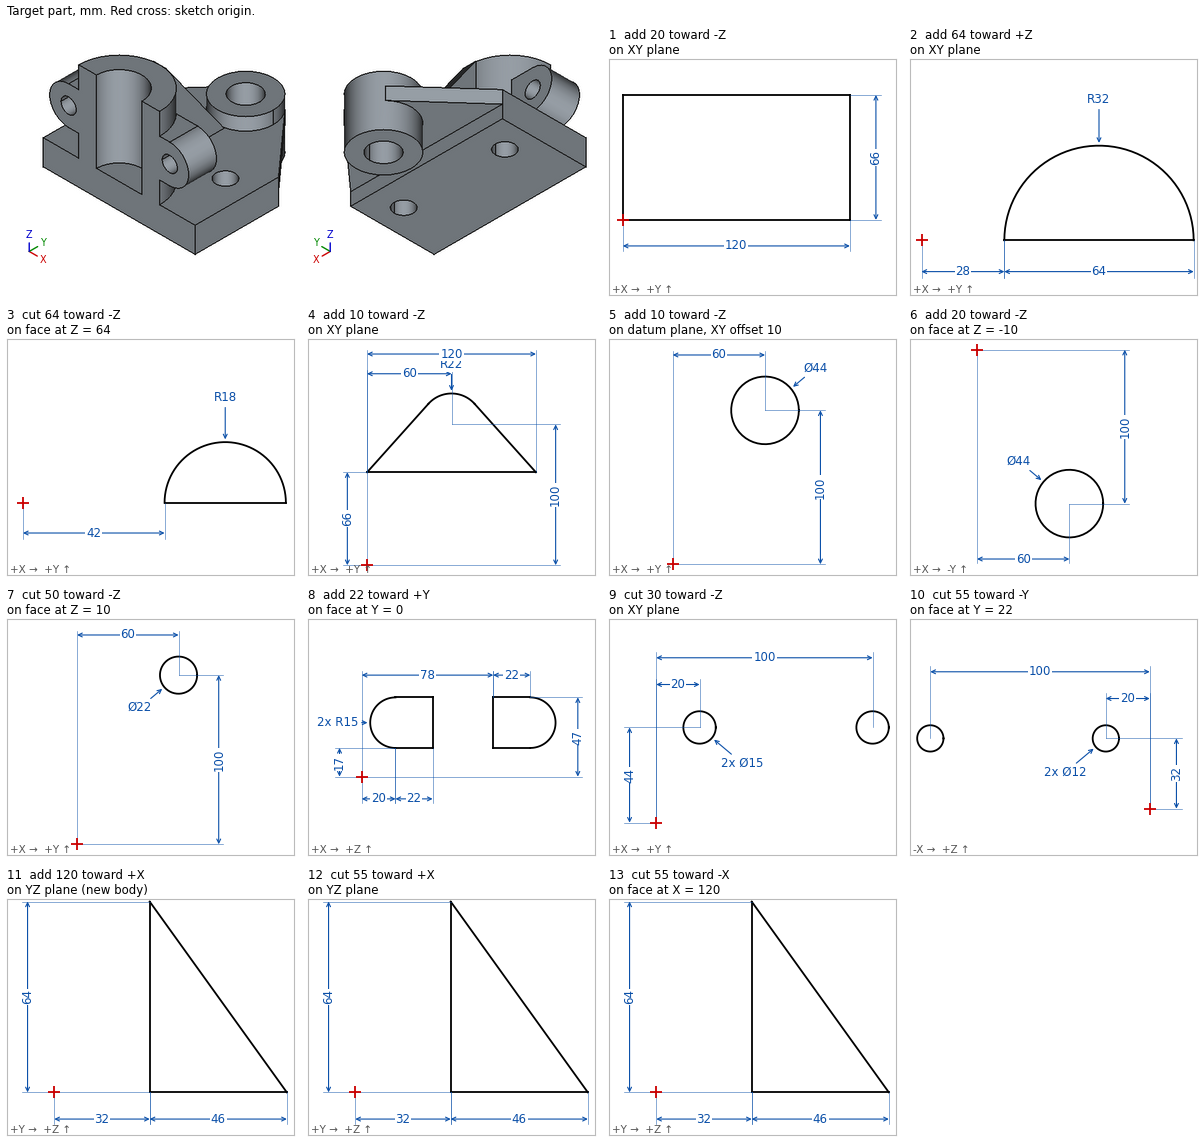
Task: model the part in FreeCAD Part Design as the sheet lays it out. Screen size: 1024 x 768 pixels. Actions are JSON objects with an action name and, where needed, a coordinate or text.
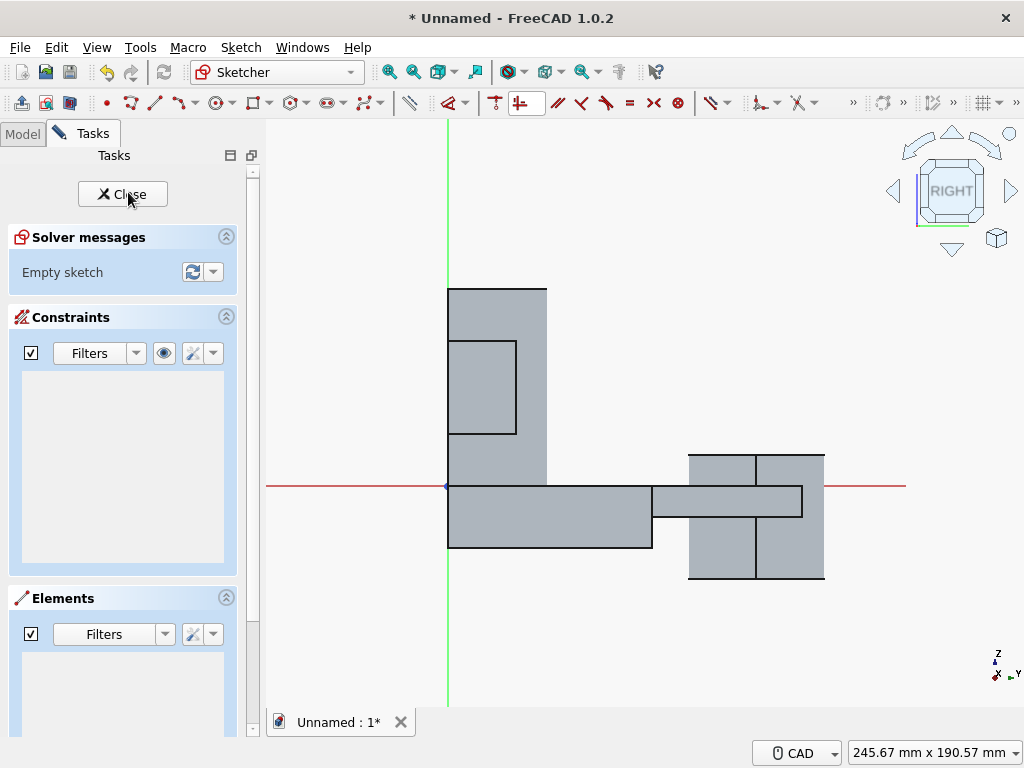
{"action": "scroll", "coordinate": [558, 356], "scroll_direction": "up", "scroll_amount": 3}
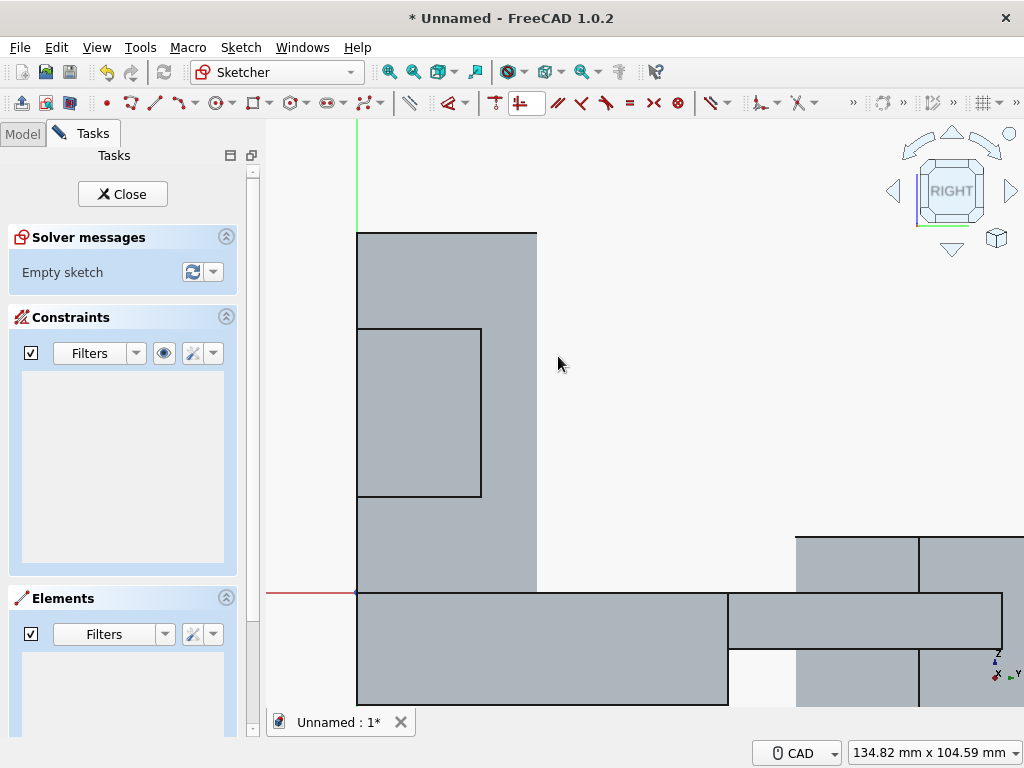
{"action": "left_click", "coordinate": [132, 104]}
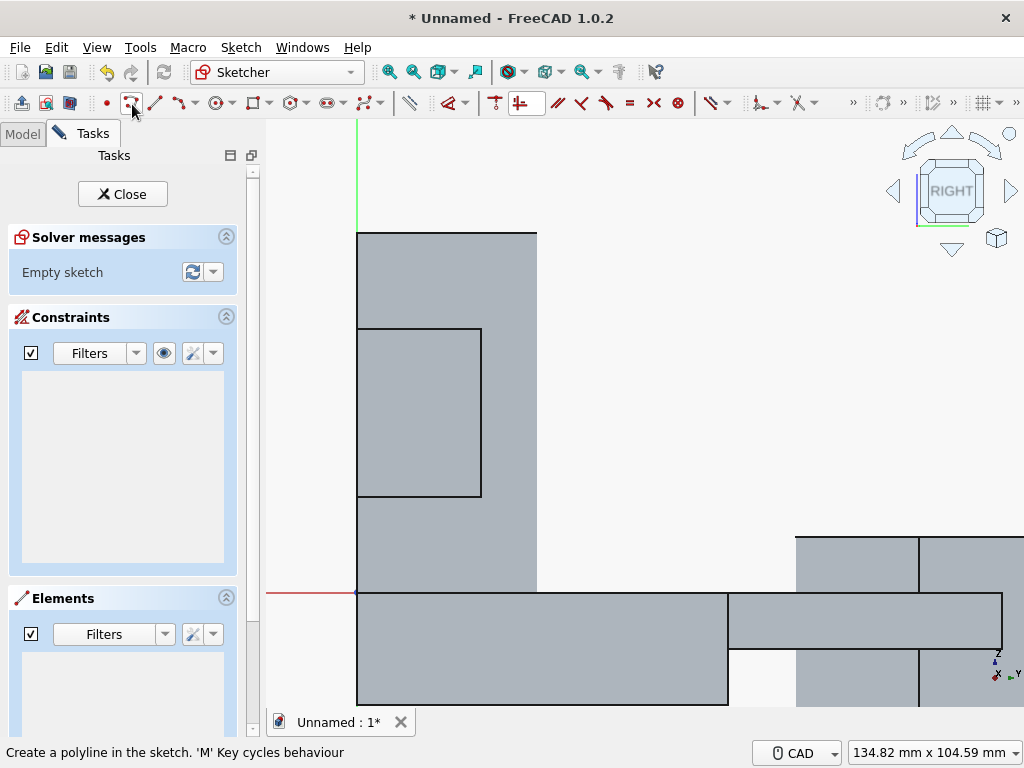
{"action": "left_click", "coordinate": [537, 593]}
{"action": "left_click", "coordinate": [537, 233]}
{"action": "left_click", "coordinate": [796, 584]}
{"action": "left_click", "coordinate": [537, 593]}
{"action": "key", "text": "Escape"}
{"action": "key", "text": "Escape"}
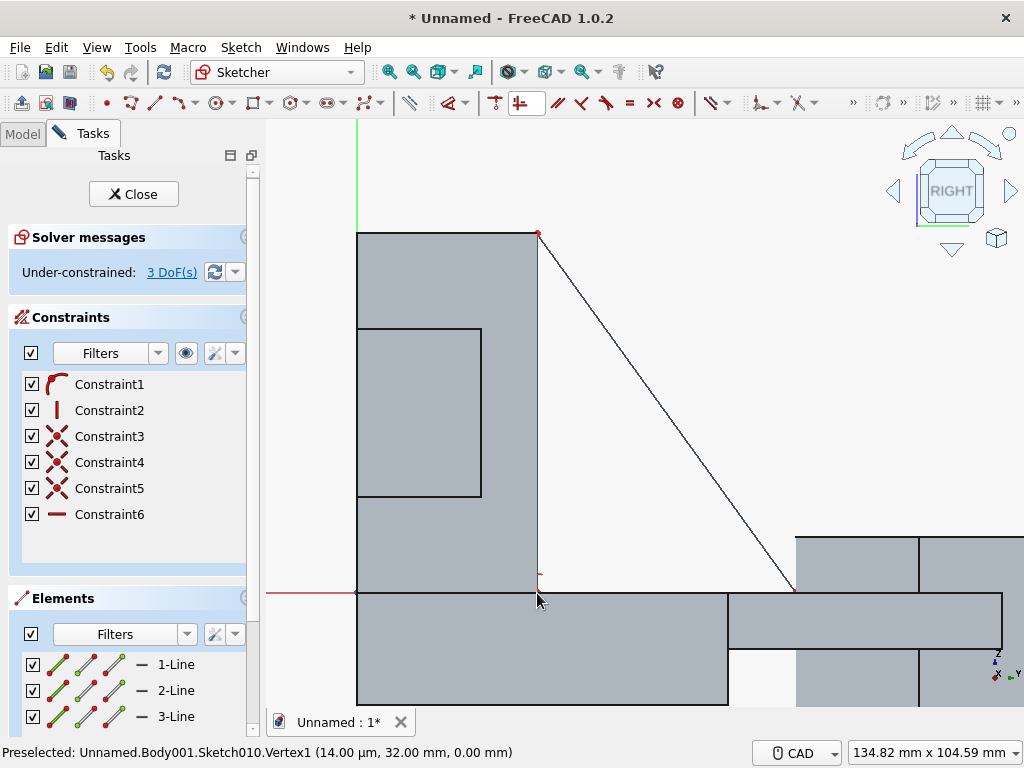
{"action": "left_click", "coordinate": [448, 104]}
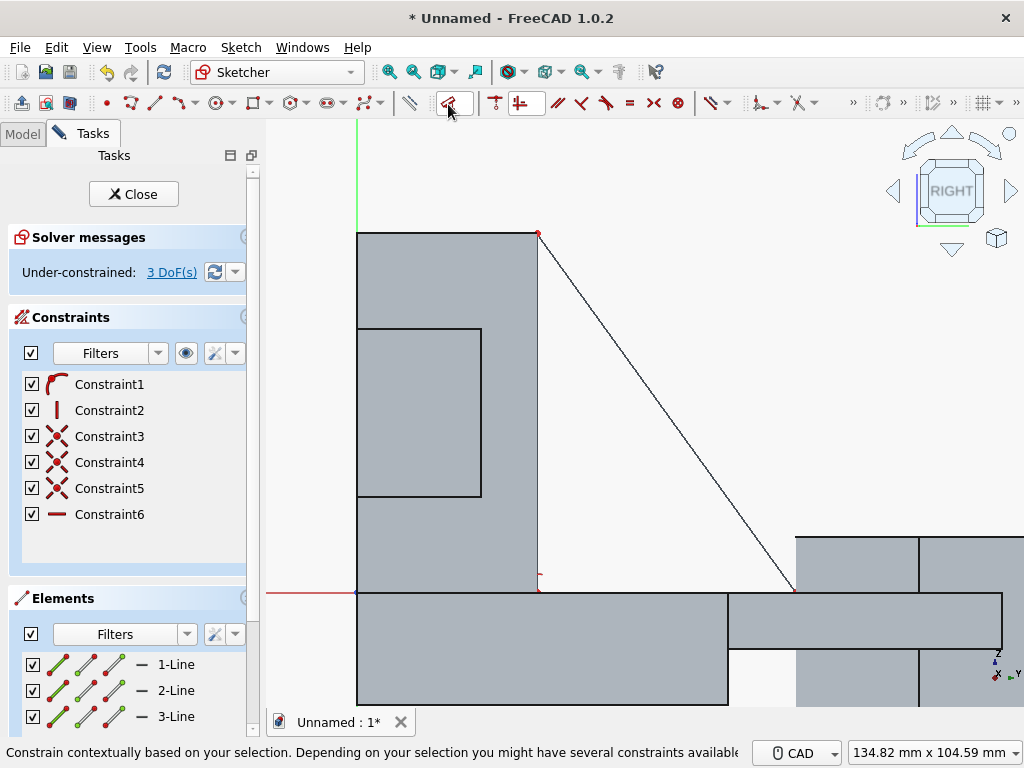
{"action": "left_click", "coordinate": [537, 485]}
{"action": "left_click", "coordinate": [503, 413]}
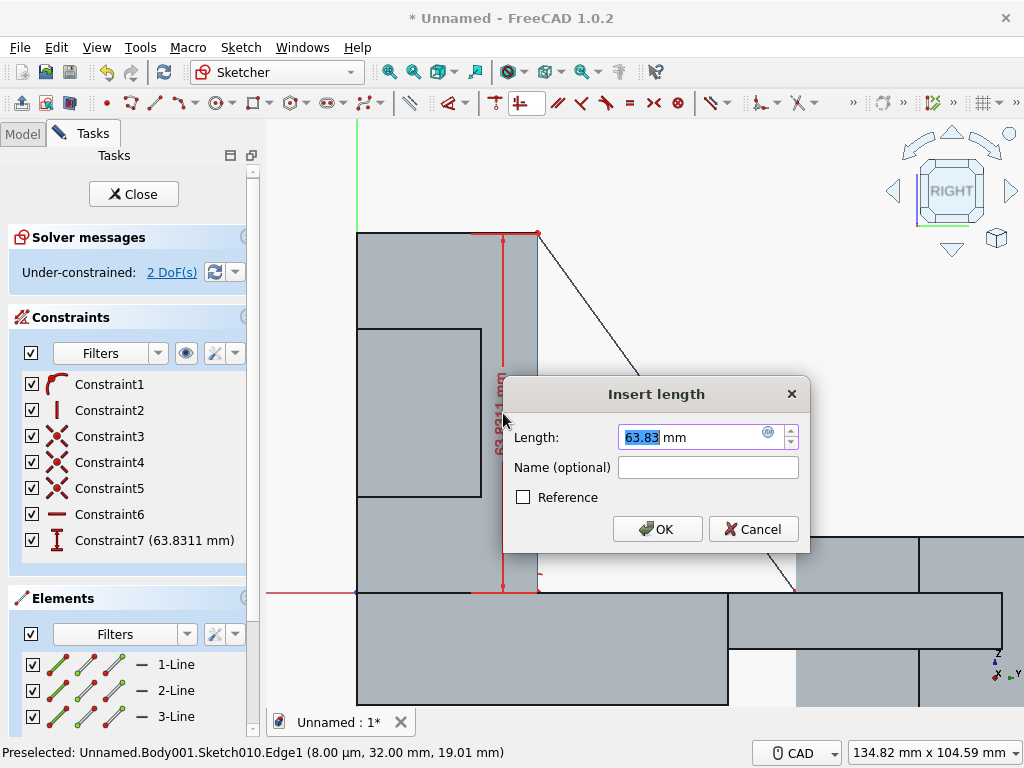
{"action": "type", "text": "64"}
{"action": "key", "text": "Return"}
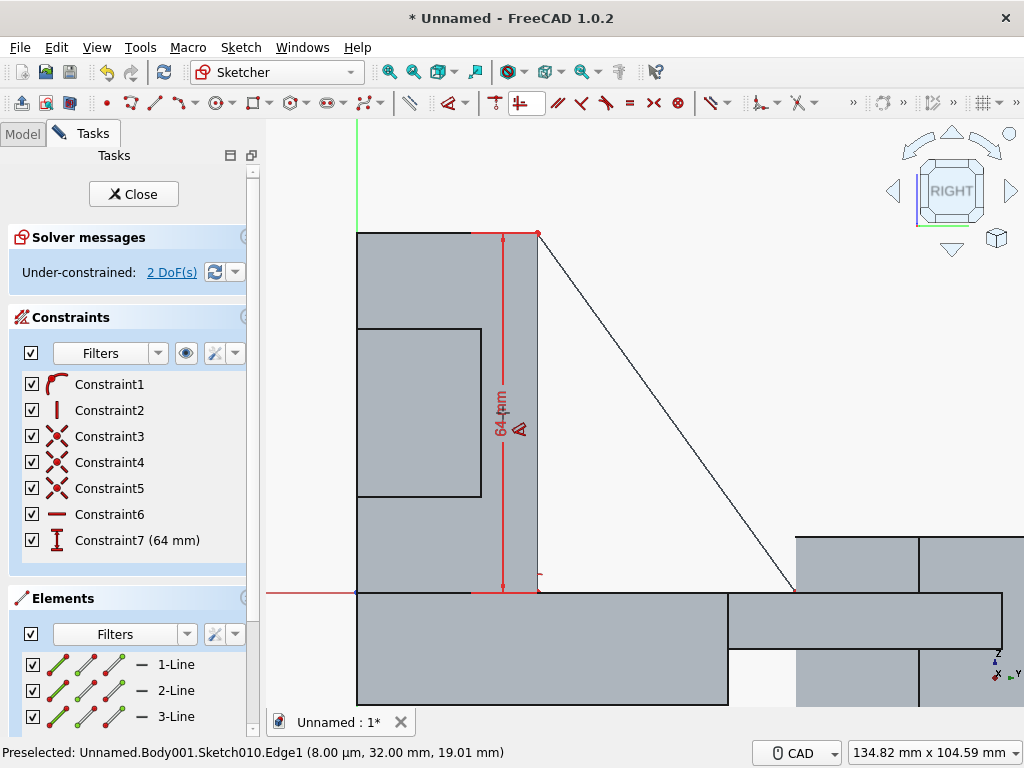
{"action": "left_click", "coordinate": [718, 593]}
{"action": "left_click", "coordinate": [666, 627]}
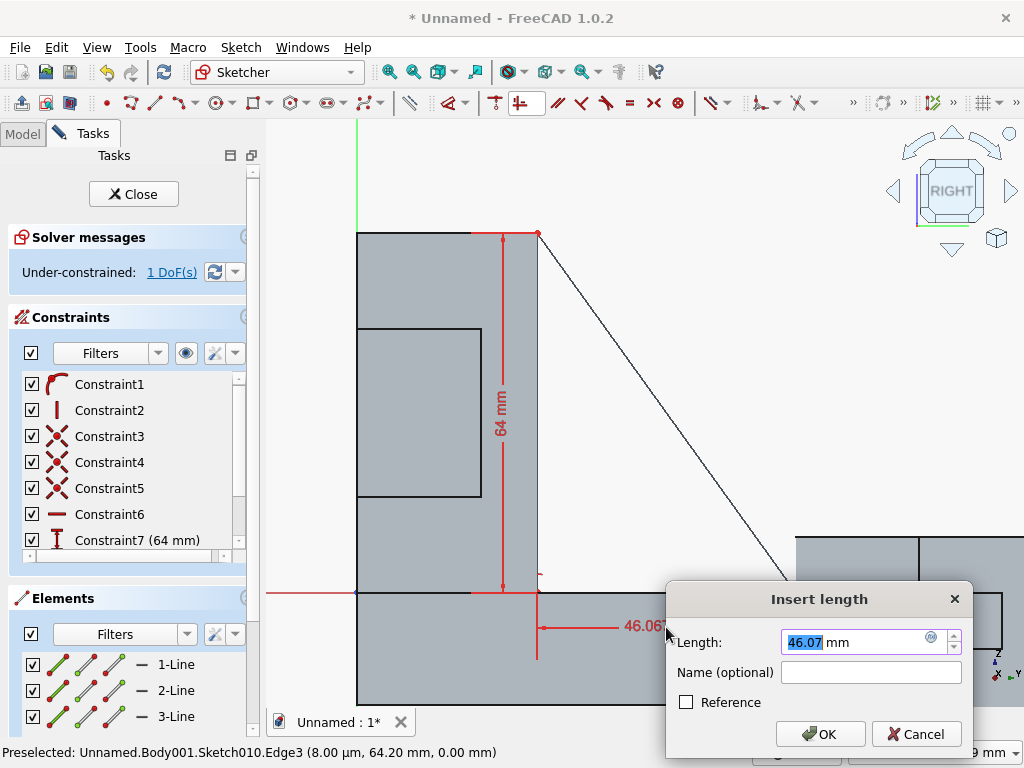
{"action": "type", "text": "46"}
{"action": "key", "text": "Return"}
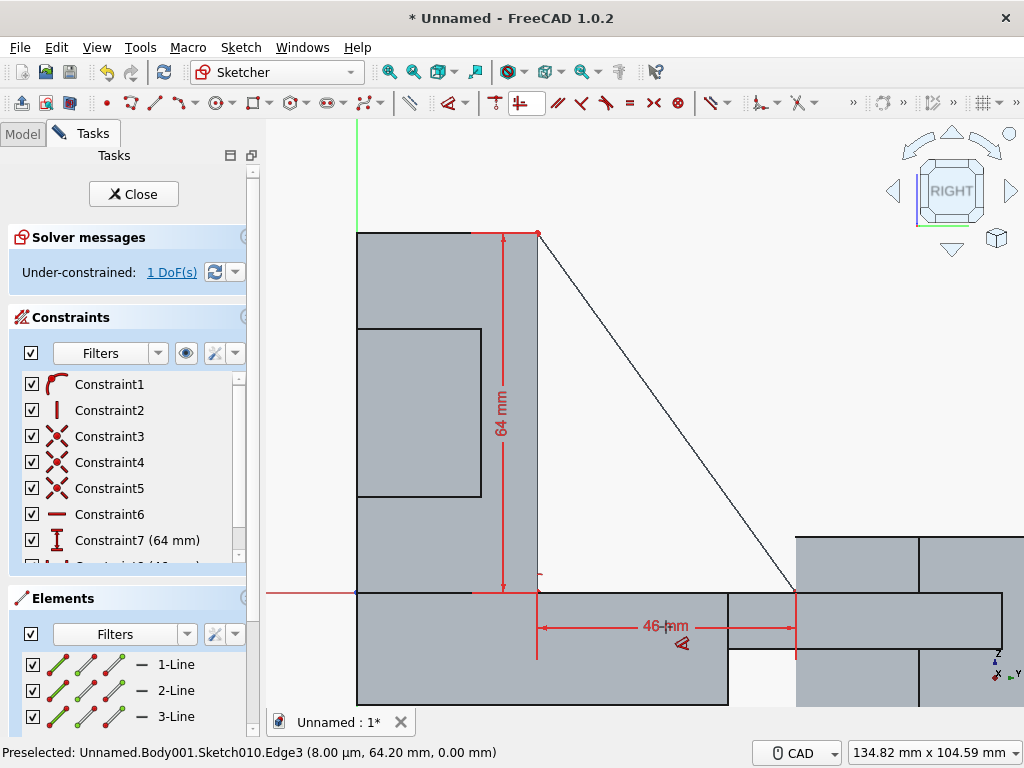
{"action": "left_click", "coordinate": [537, 593]}
{"action": "left_click", "coordinate": [447, 627]}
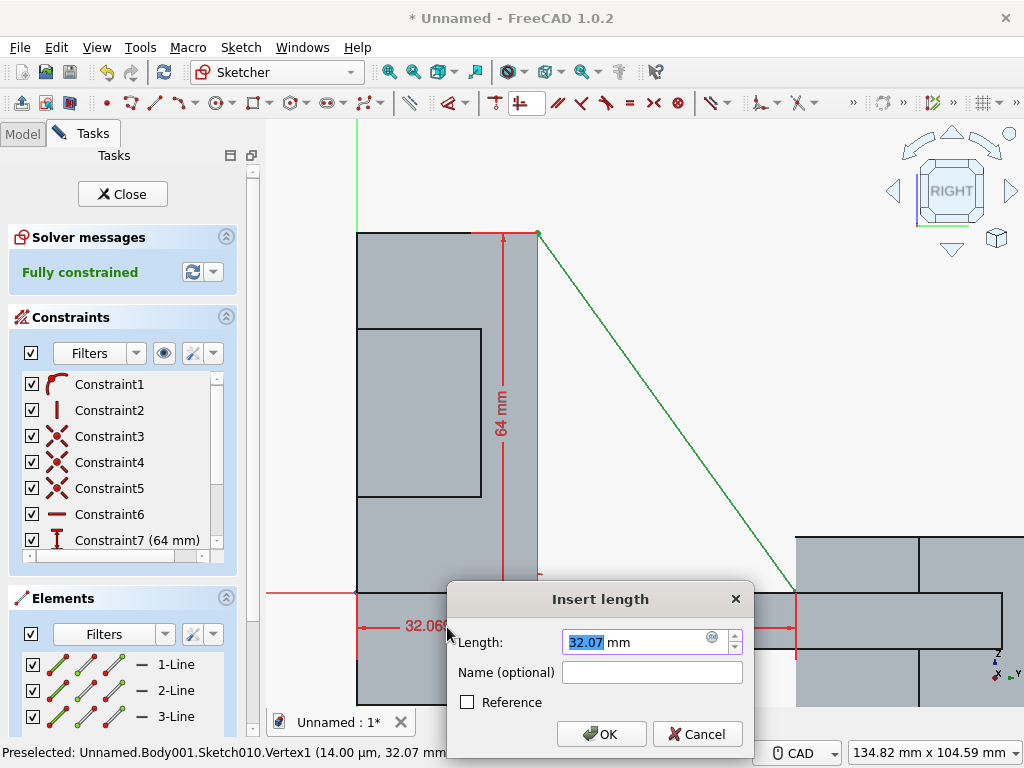
{"action": "type", "text": "32"}
{"action": "key", "text": "Return"}
{"action": "key", "text": "Escape"}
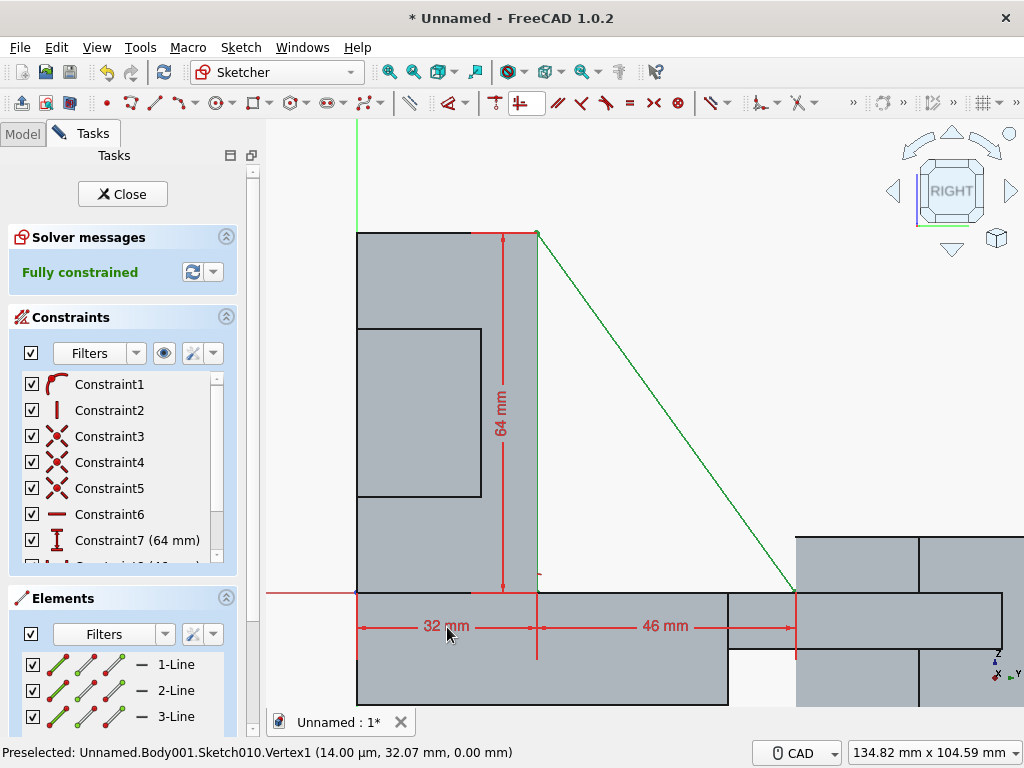
{"action": "left_click", "coordinate": [123, 194]}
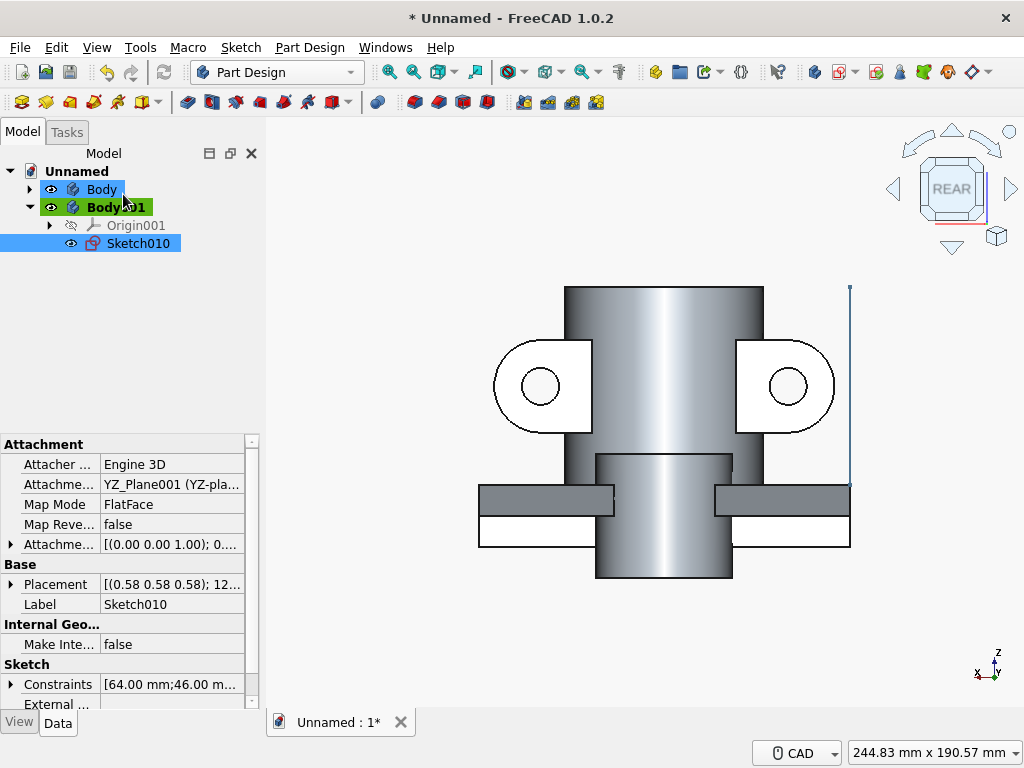
{"action": "left_click", "coordinate": [22, 102]}